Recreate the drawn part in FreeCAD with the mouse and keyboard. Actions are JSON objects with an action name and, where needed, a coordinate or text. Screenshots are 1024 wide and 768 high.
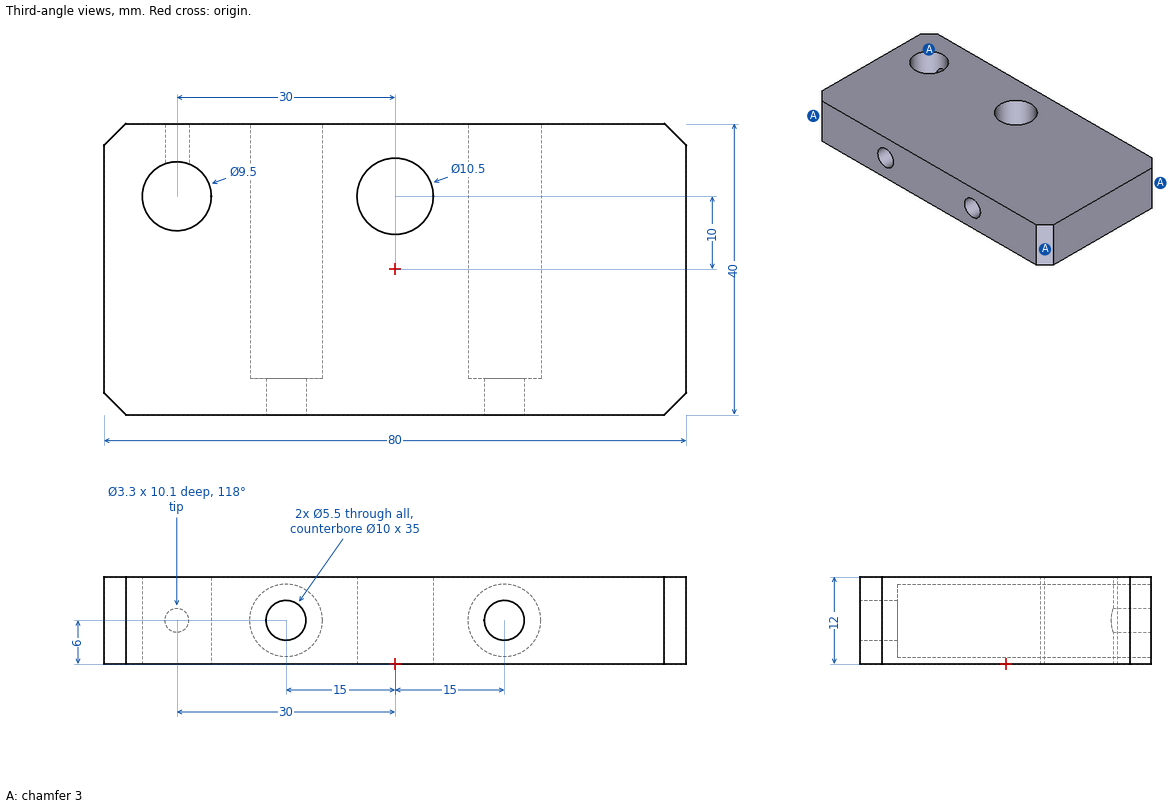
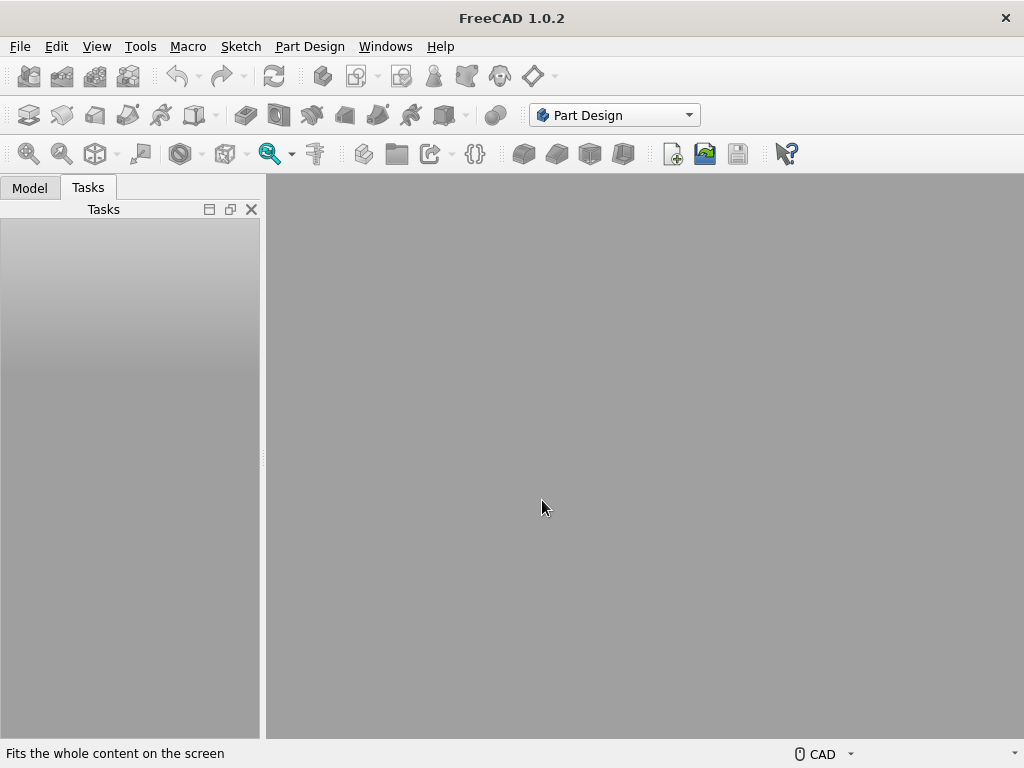
{"action": "key", "text": "ctrl+n"}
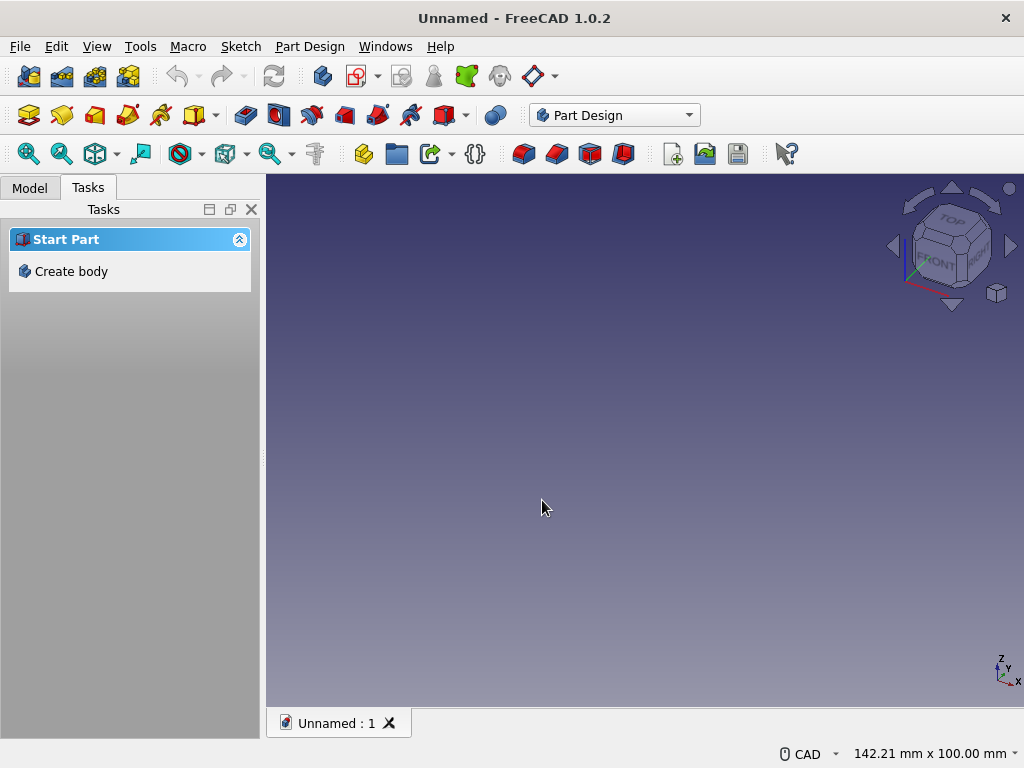
{"action": "left_click", "coordinate": [356, 76]}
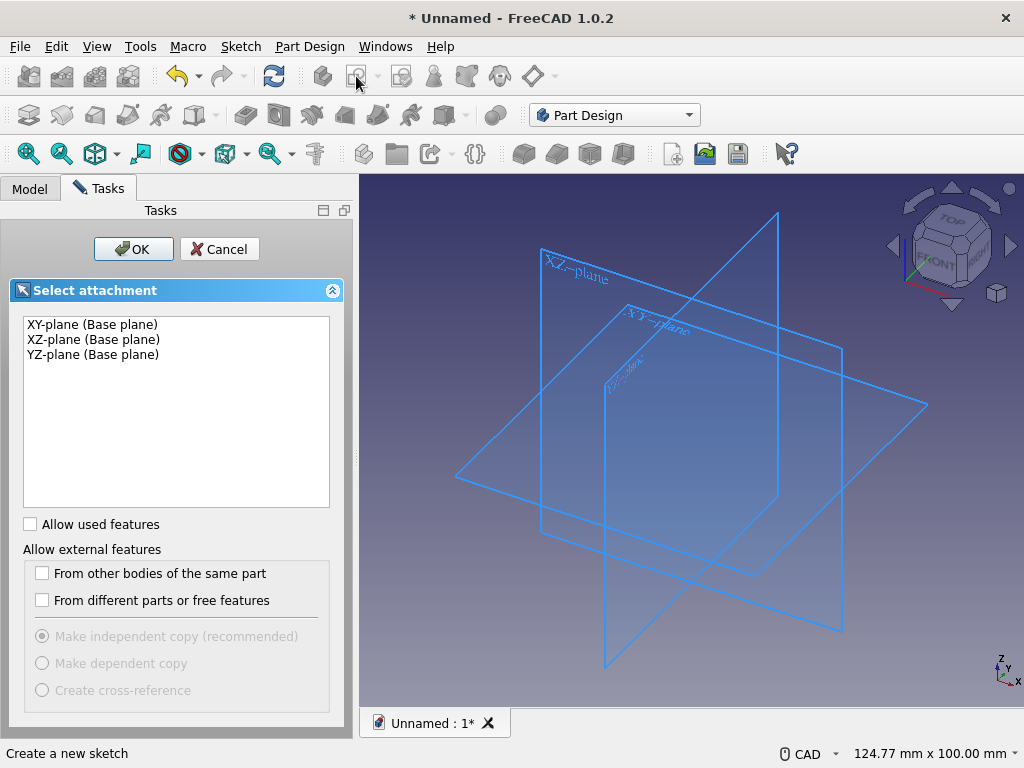
{"action": "left_click", "coordinate": [84, 324]}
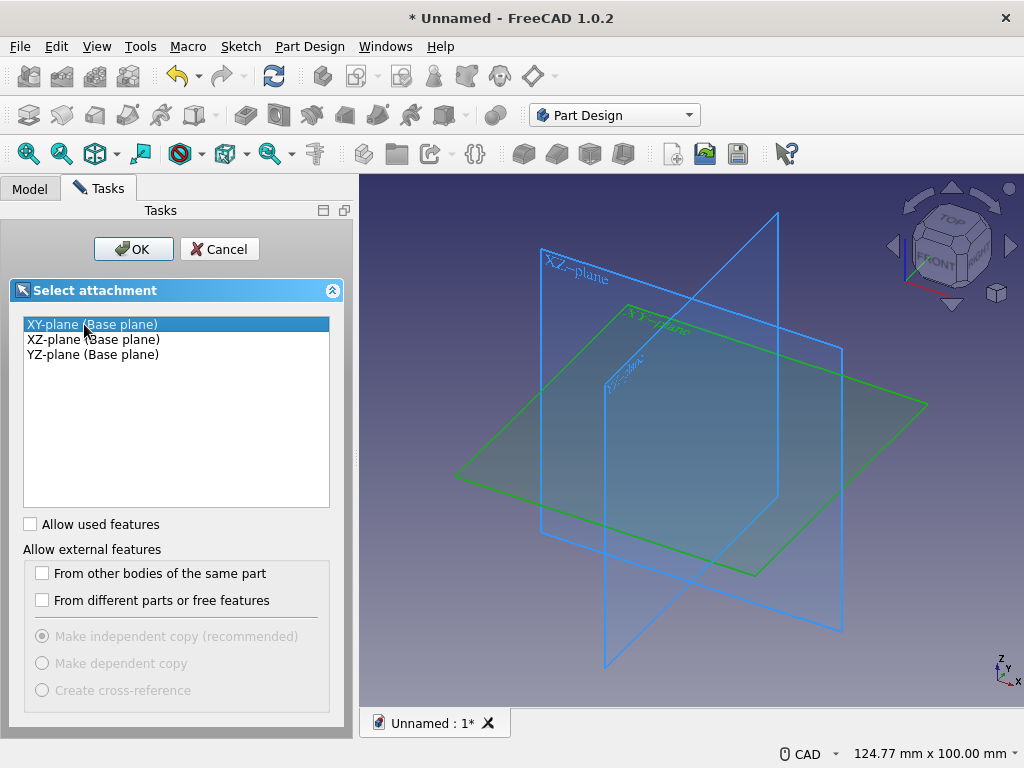
{"action": "left_click", "coordinate": [134, 249]}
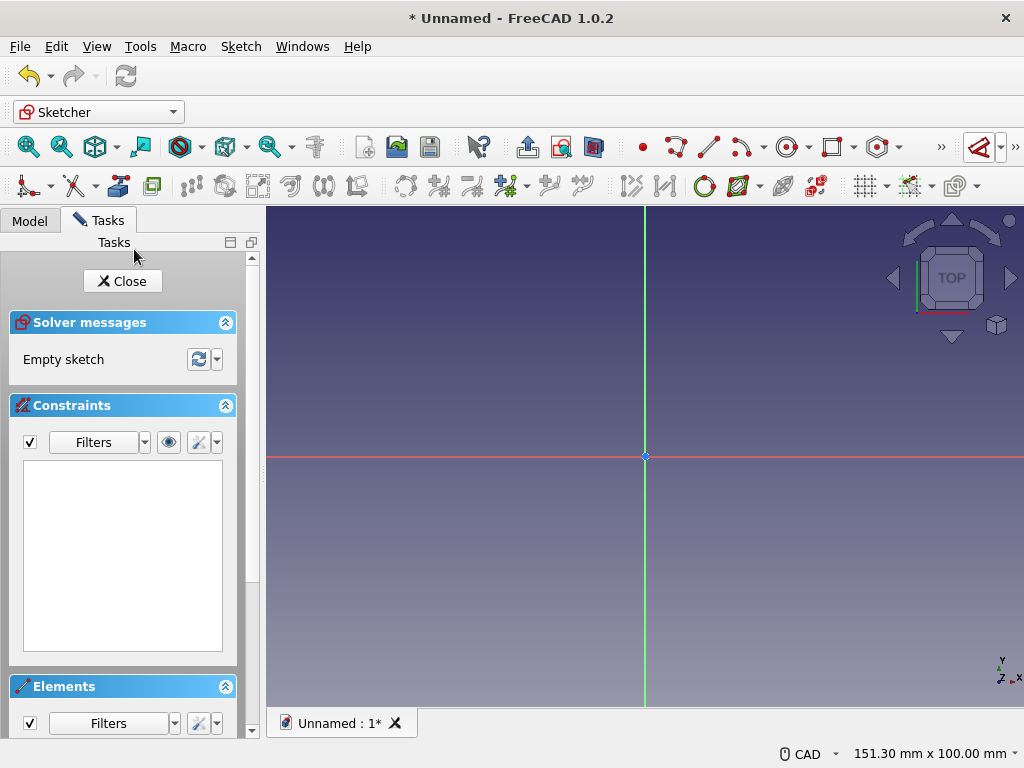
{"action": "scroll", "coordinate": [294, 456], "scroll_direction": "down", "scroll_amount": 1}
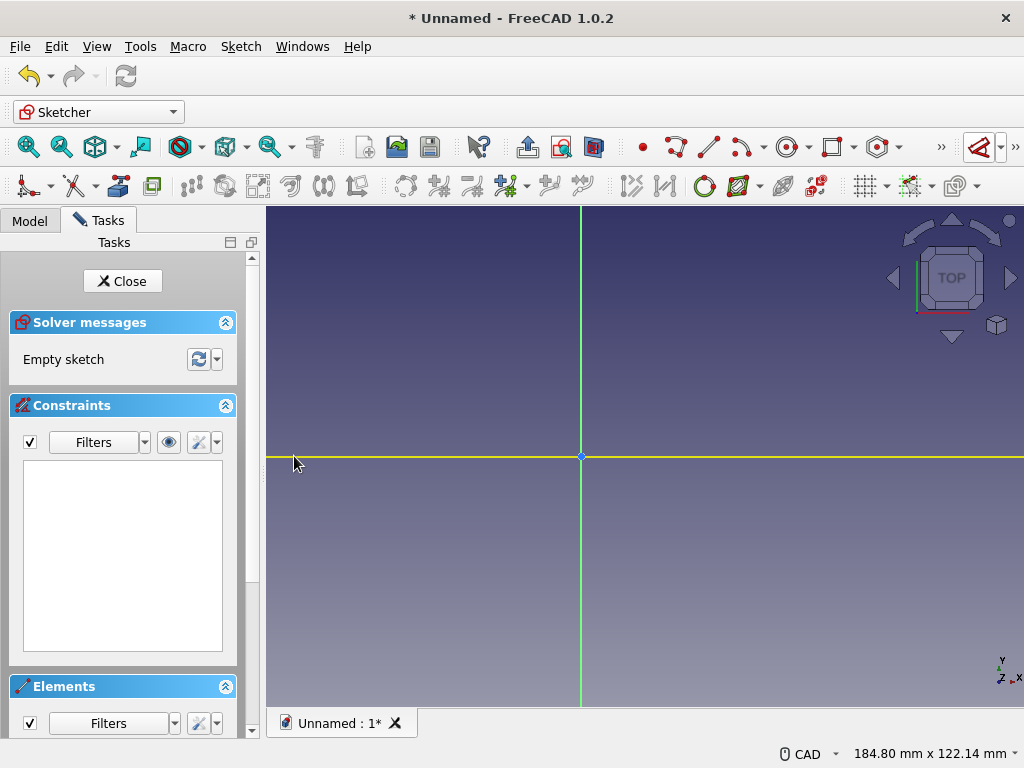
{"action": "key", "text": "g v"}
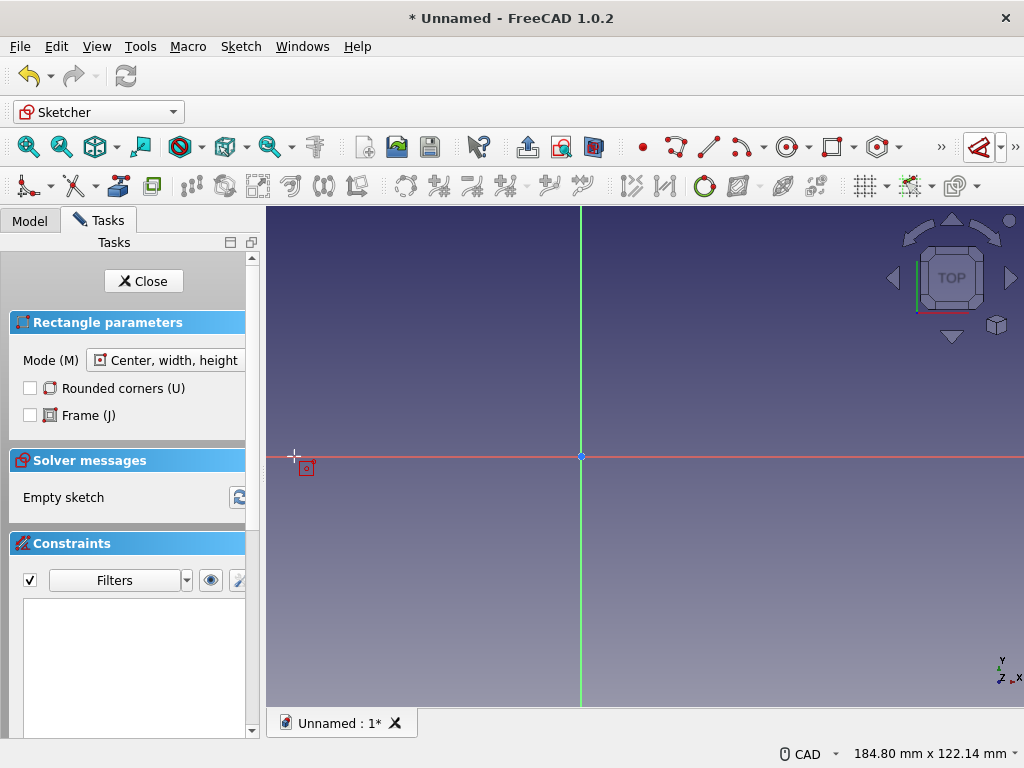
{"action": "left_click", "coordinate": [581, 456]}
{"action": "left_click", "coordinate": [745, 374]}
{"action": "key", "text": "Escape"}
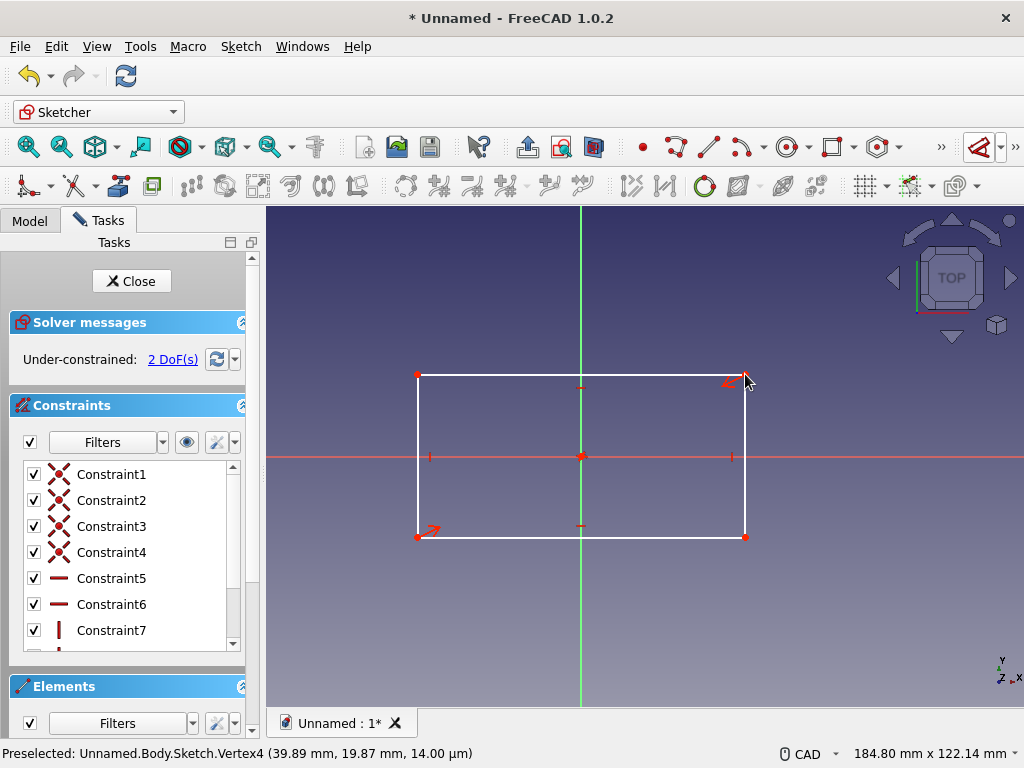
{"action": "left_click", "coordinate": [516, 538]}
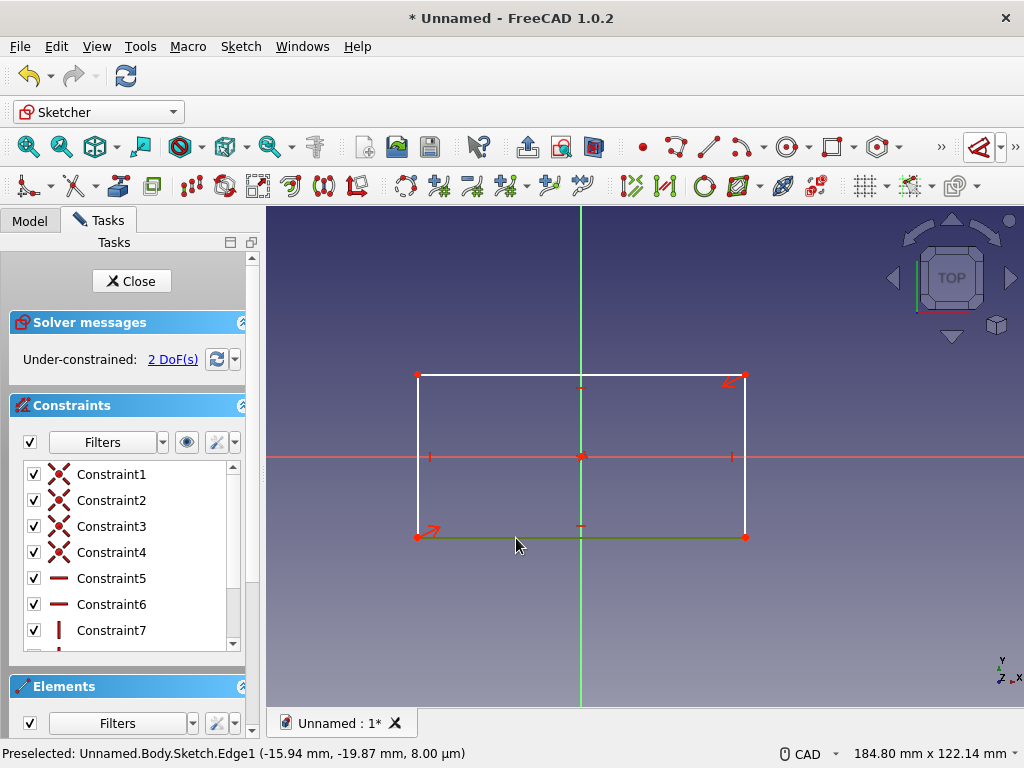
{"action": "key", "text": "l"}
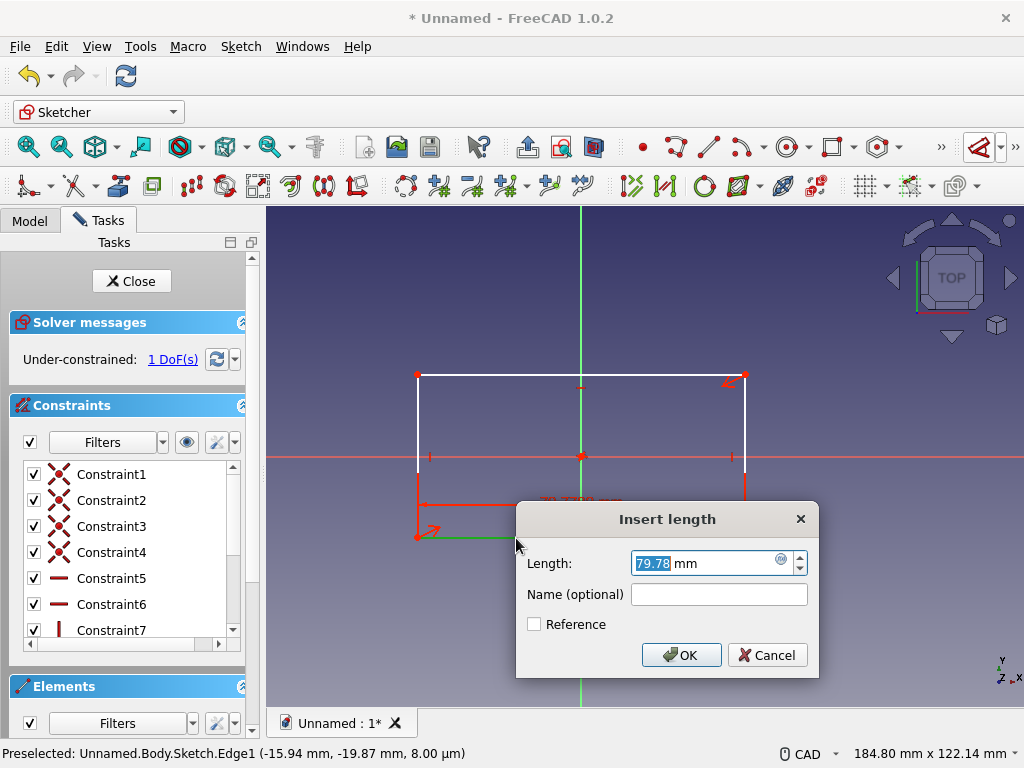
{"action": "type", "text": "80"}
{"action": "key", "text": "Return"}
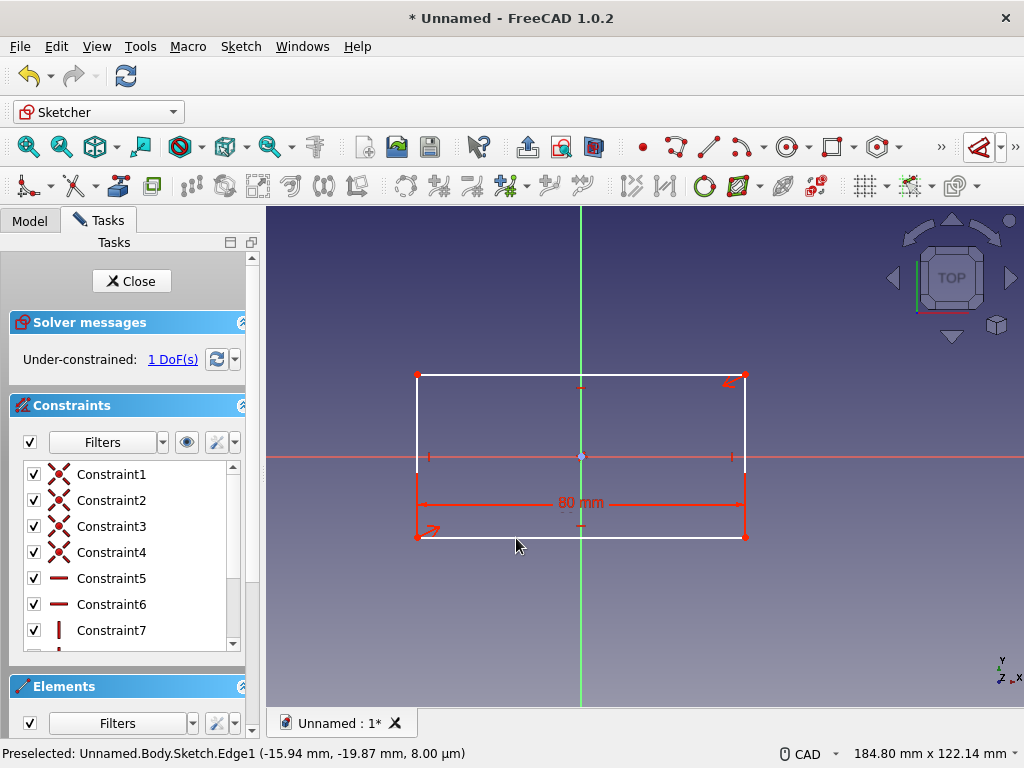
{"action": "left_click", "coordinate": [745, 489]}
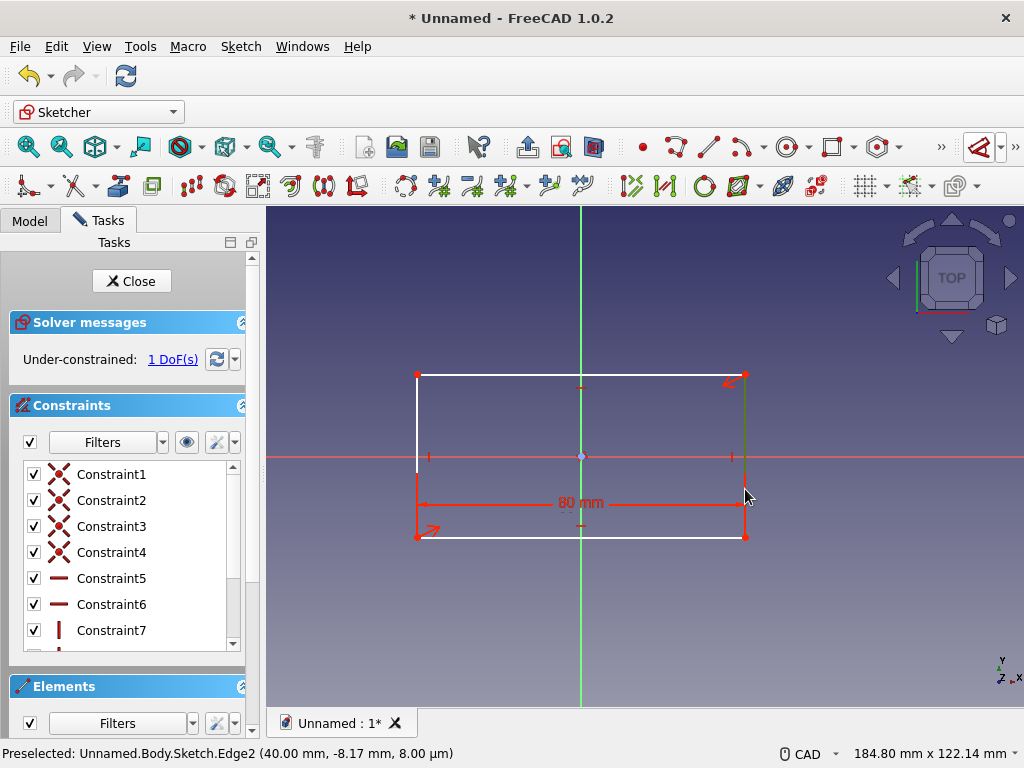
{"action": "key", "text": "i"}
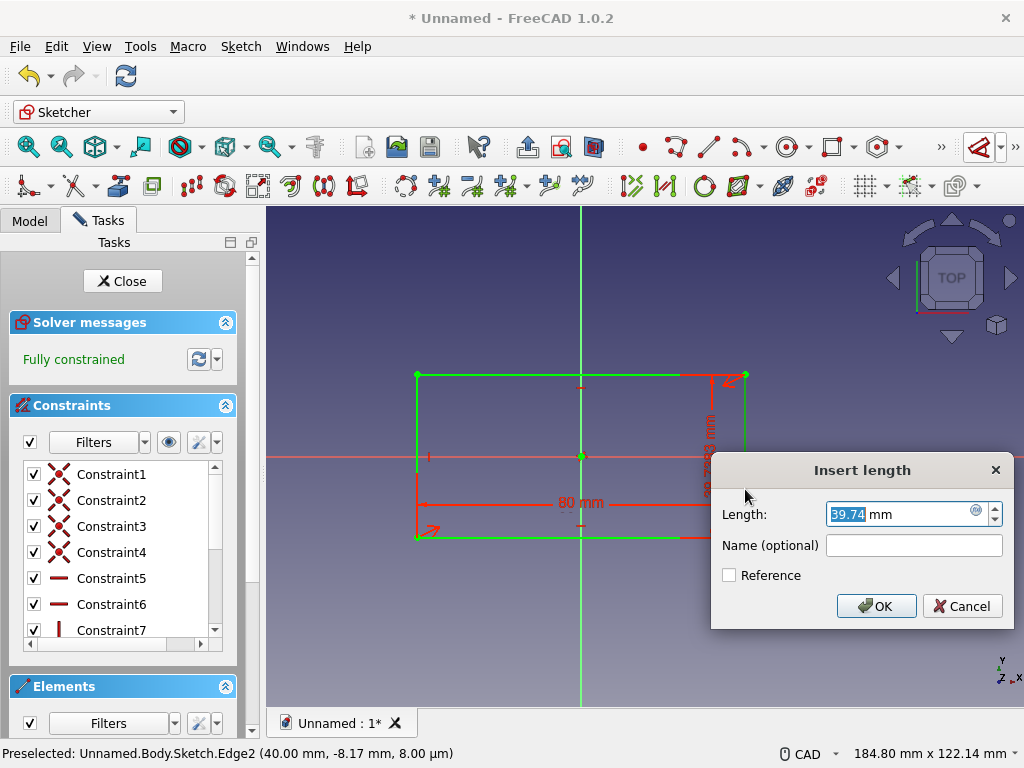
{"action": "type", "text": "40"}
{"action": "key", "text": "Return"}